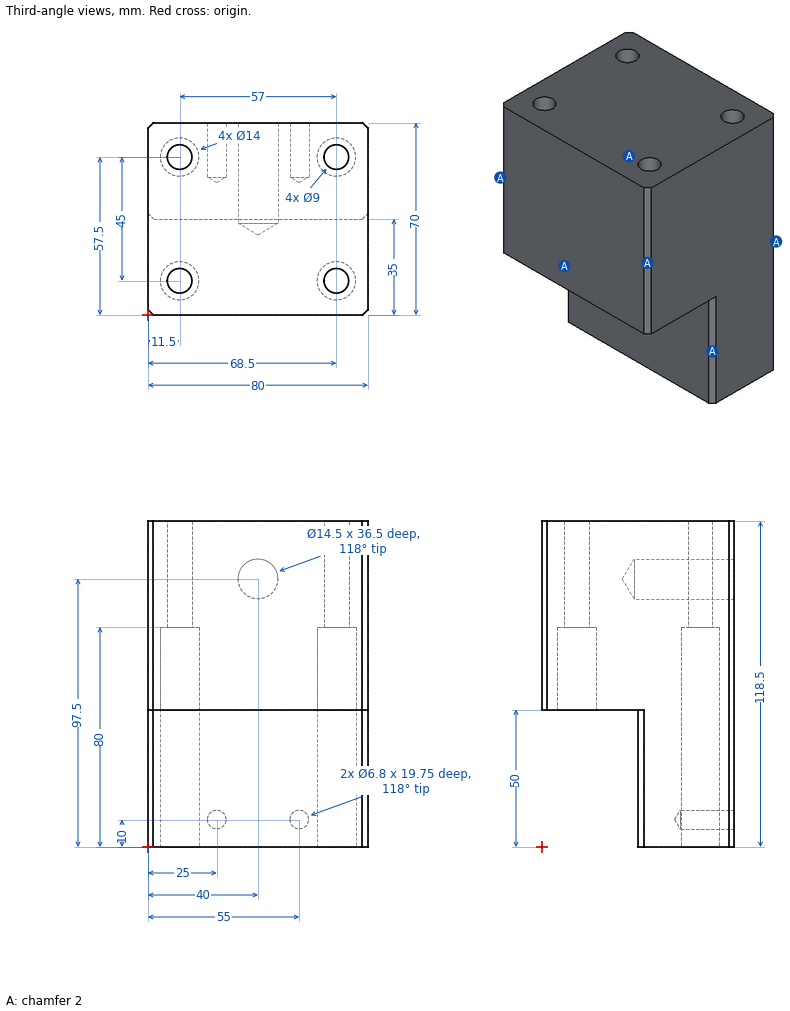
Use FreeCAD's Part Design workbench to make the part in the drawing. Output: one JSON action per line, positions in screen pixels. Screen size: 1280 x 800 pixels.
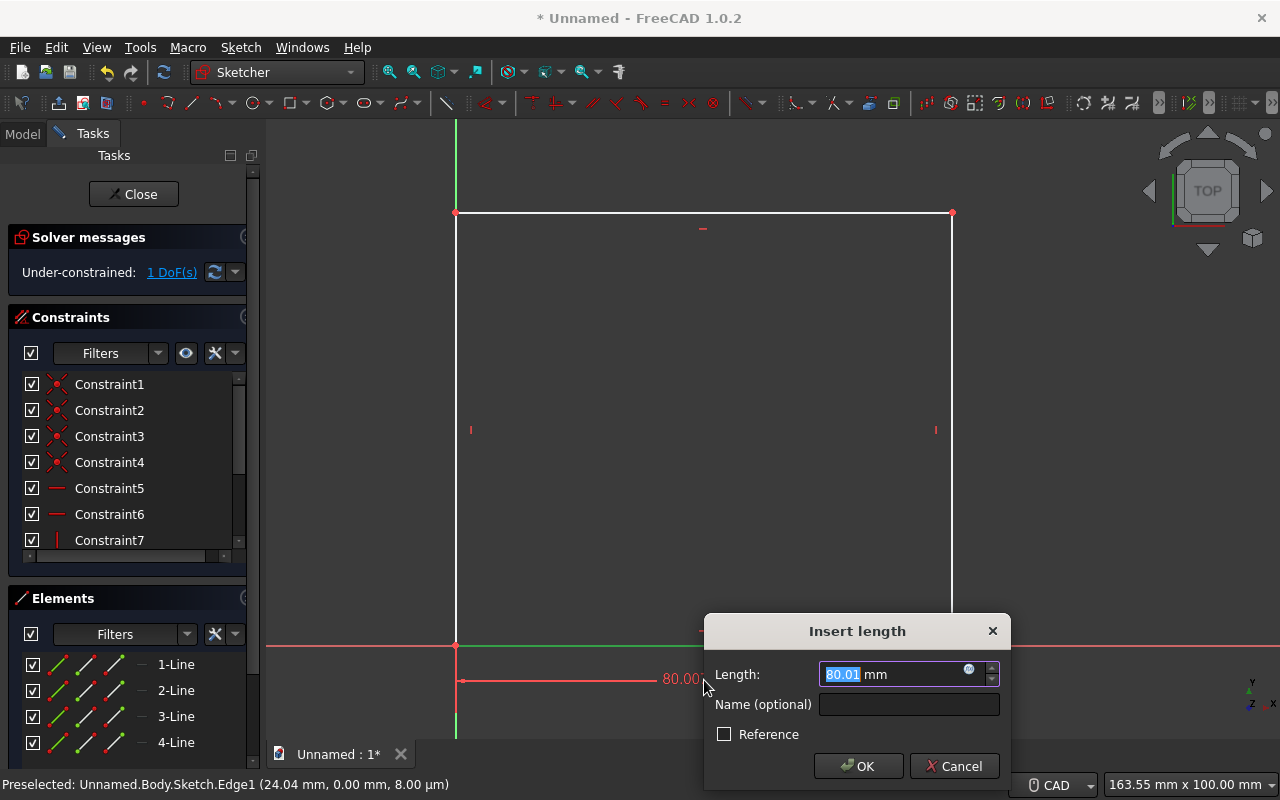
{"action": "type", "text": "80"}
{"action": "key", "text": "Return"}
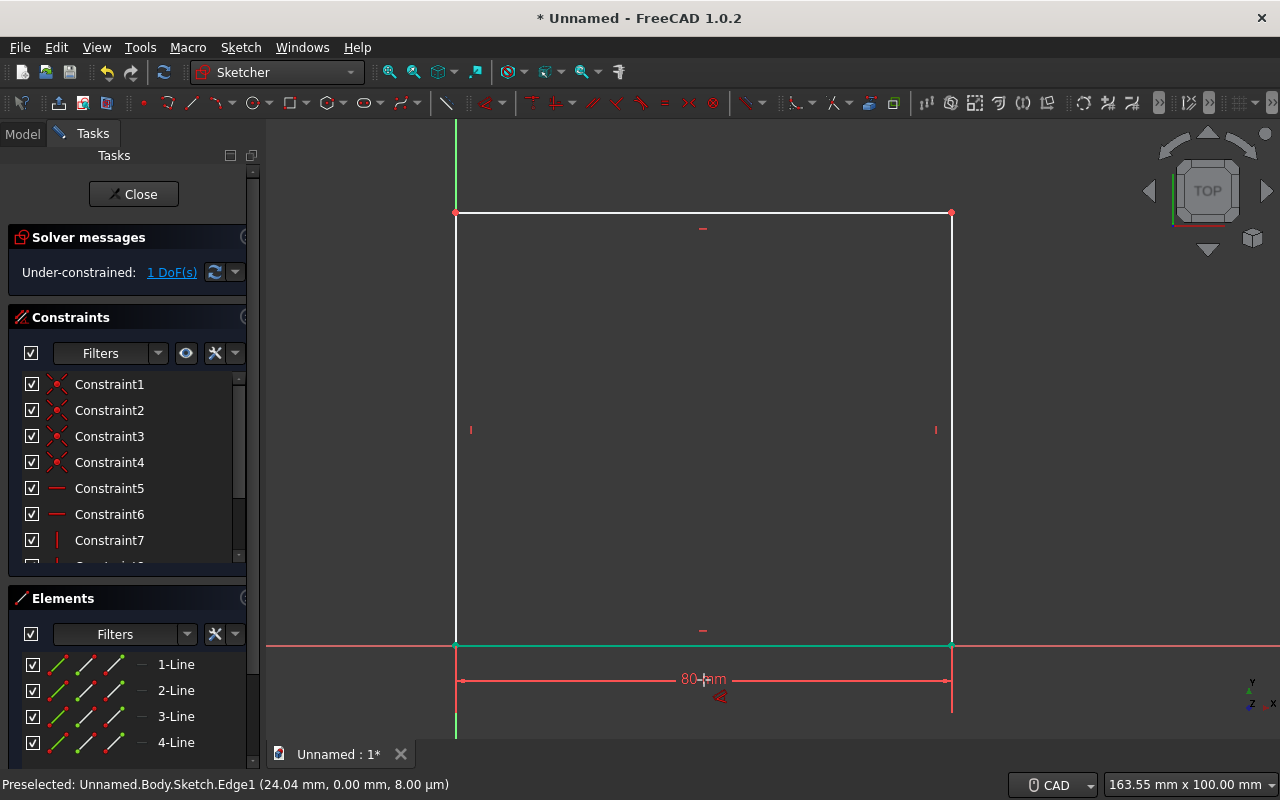
{"action": "left_click", "coordinate": [952, 516]}
{"action": "left_click", "coordinate": [986, 429]}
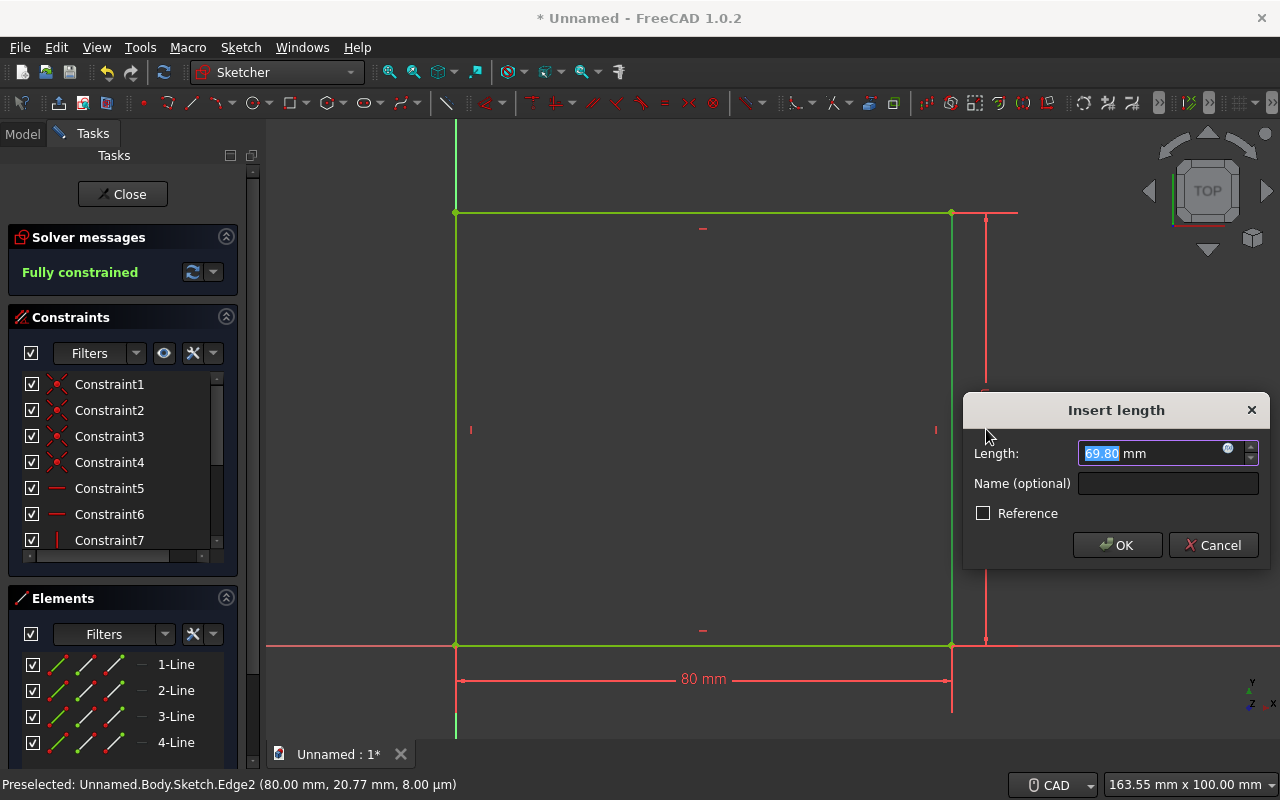
{"action": "type", "text": "70"}
{"action": "key", "text": "Return"}
{"action": "key", "text": "Escape"}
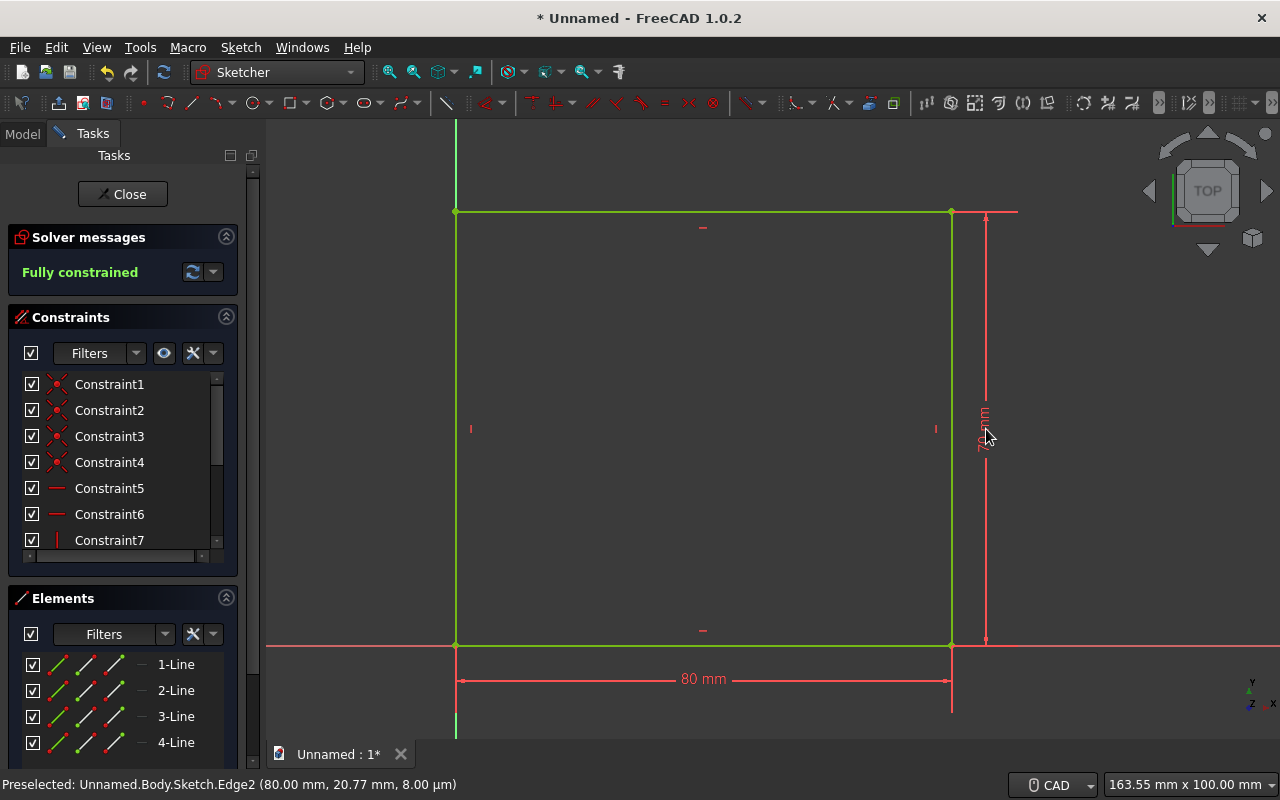
{"action": "left_click", "coordinate": [123, 194]}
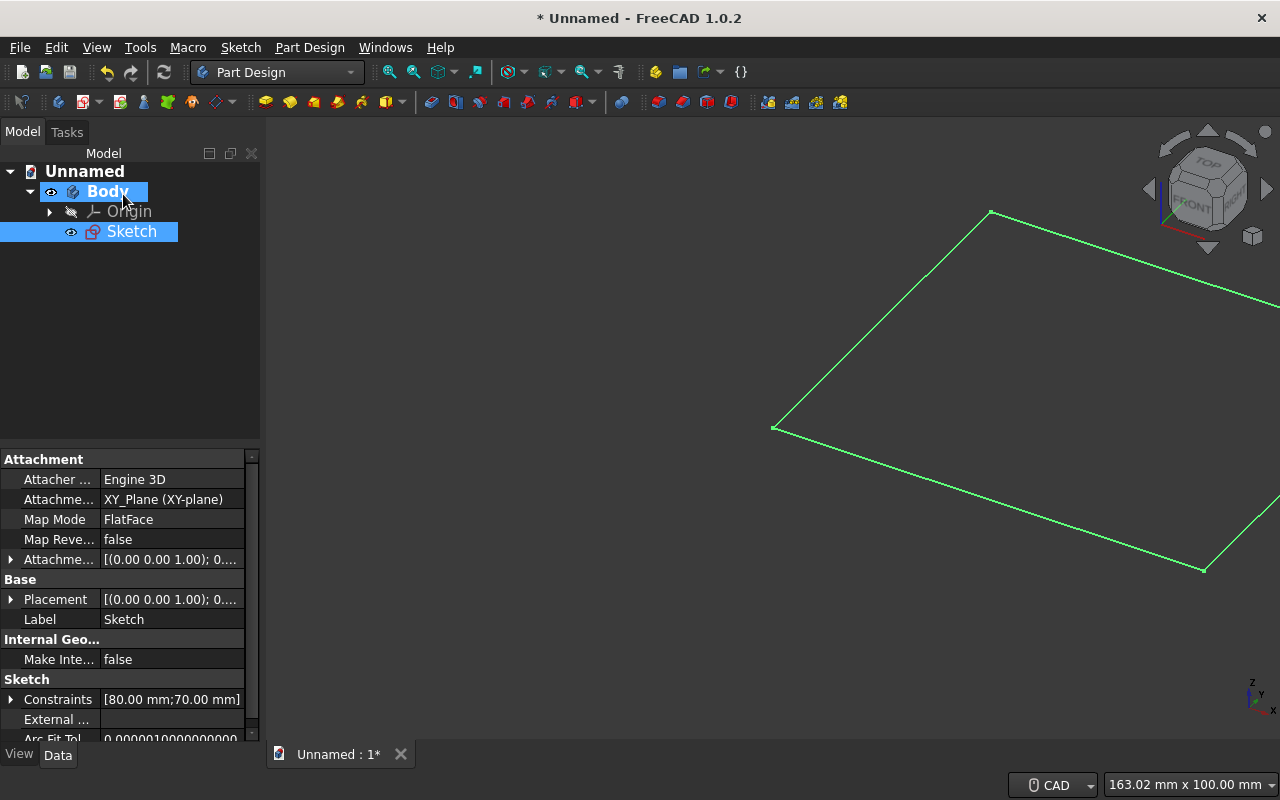
{"action": "left_click", "coordinate": [266, 102]}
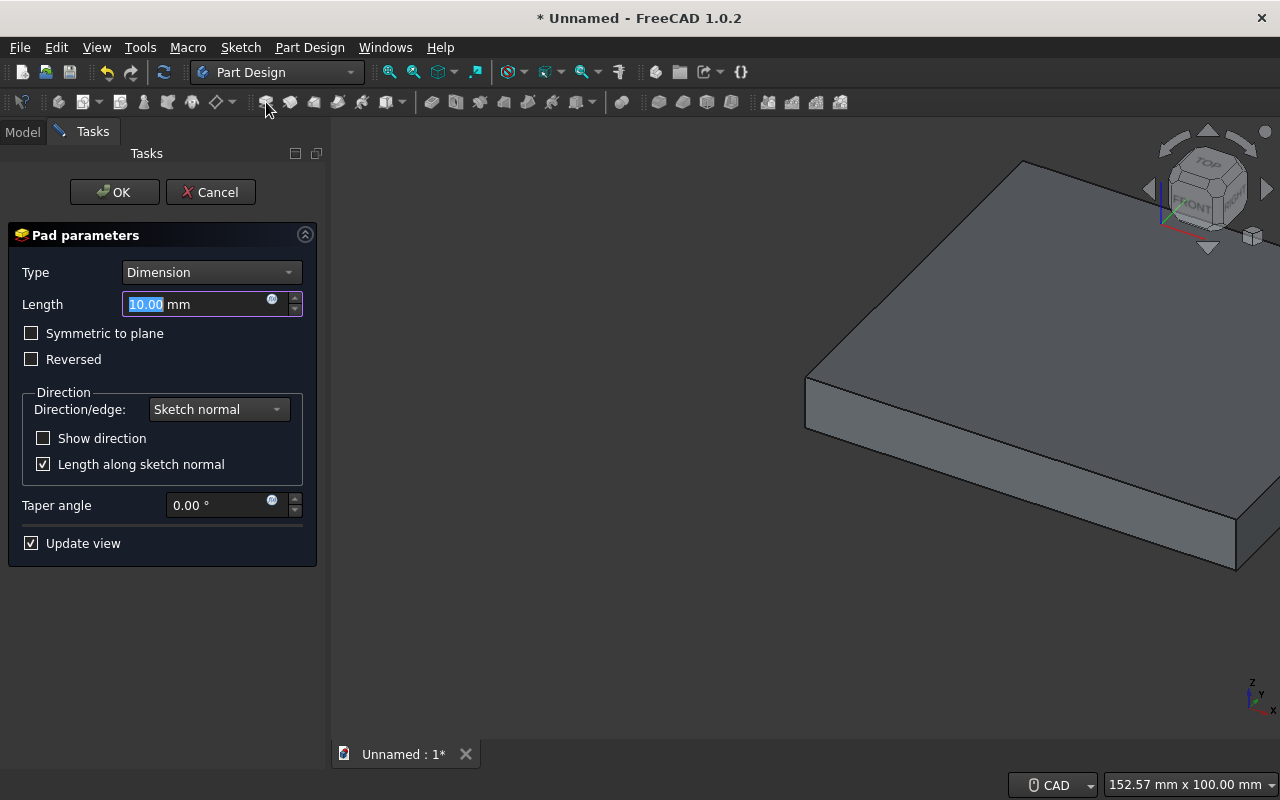
{"action": "type", "text": "118.5"}
{"action": "key", "text": "Tab"}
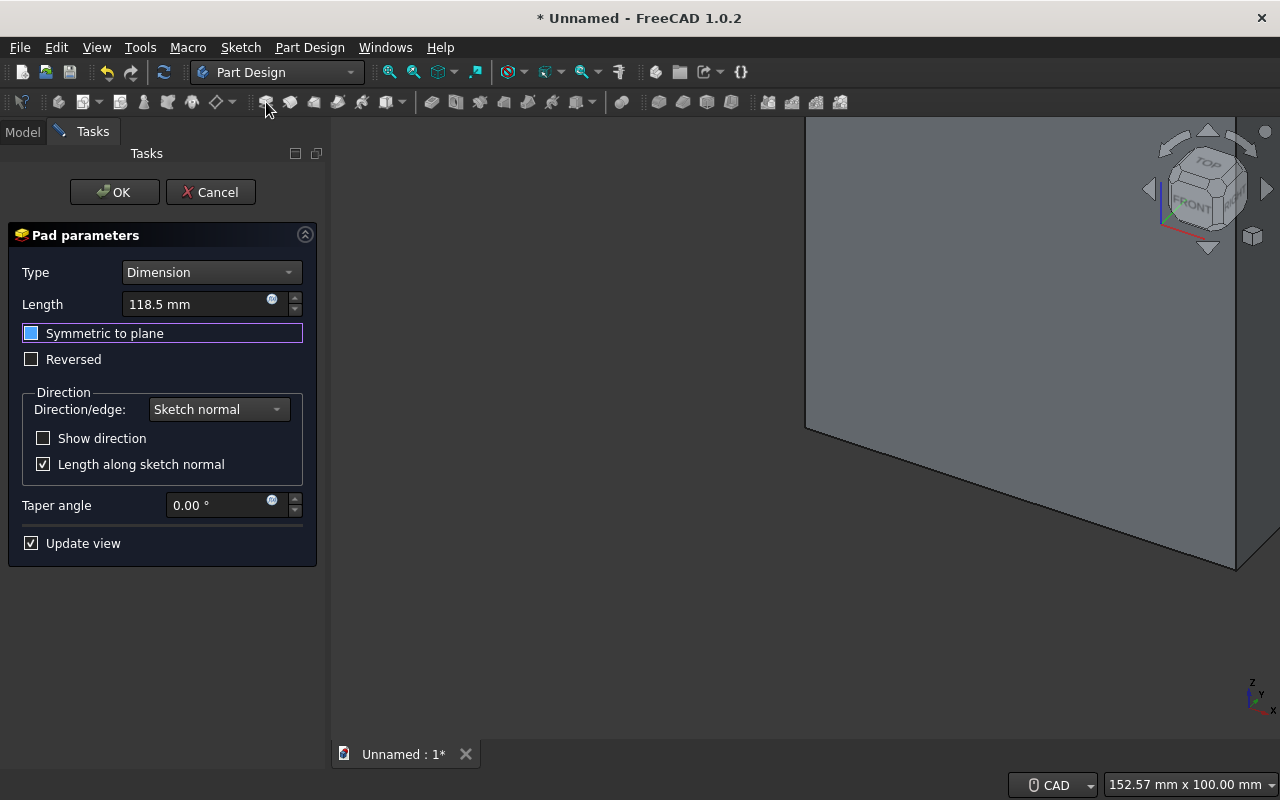
{"action": "left_click", "coordinate": [115, 192]}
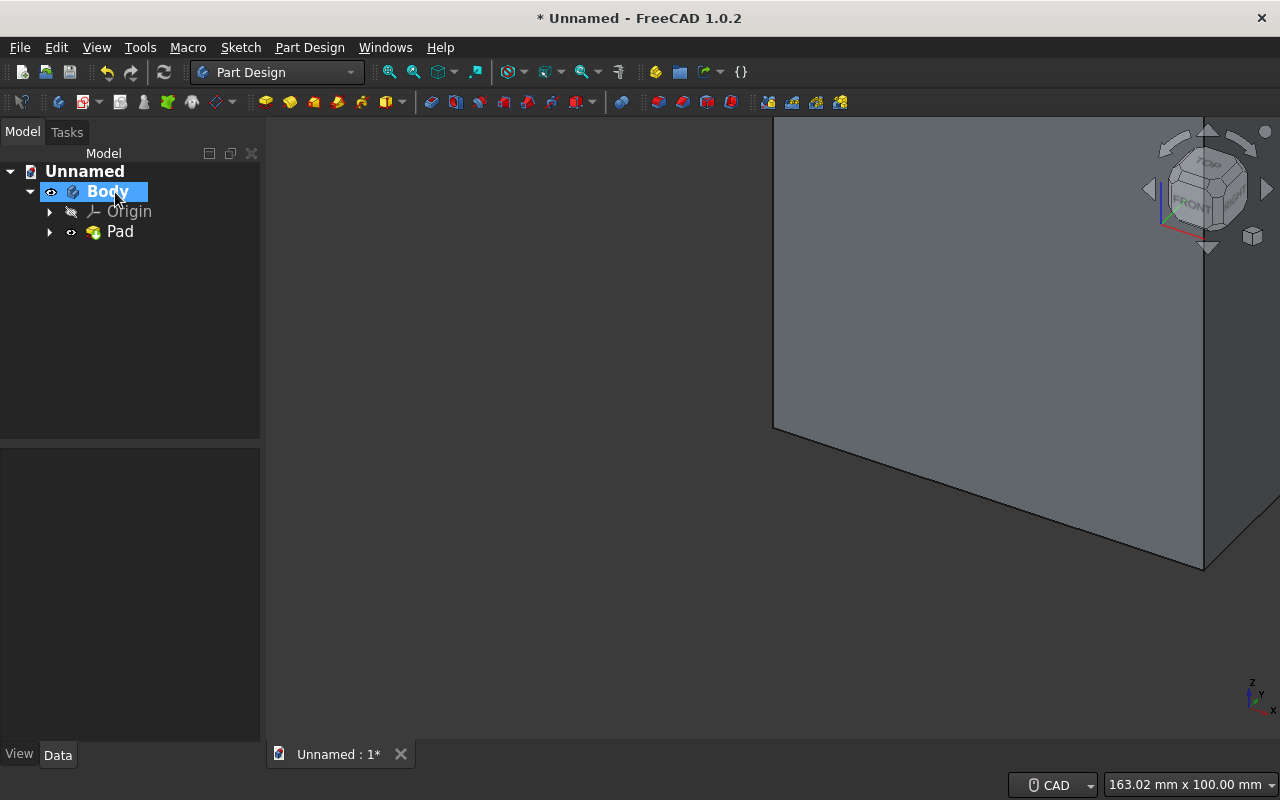
{"action": "key", "text": "v f"}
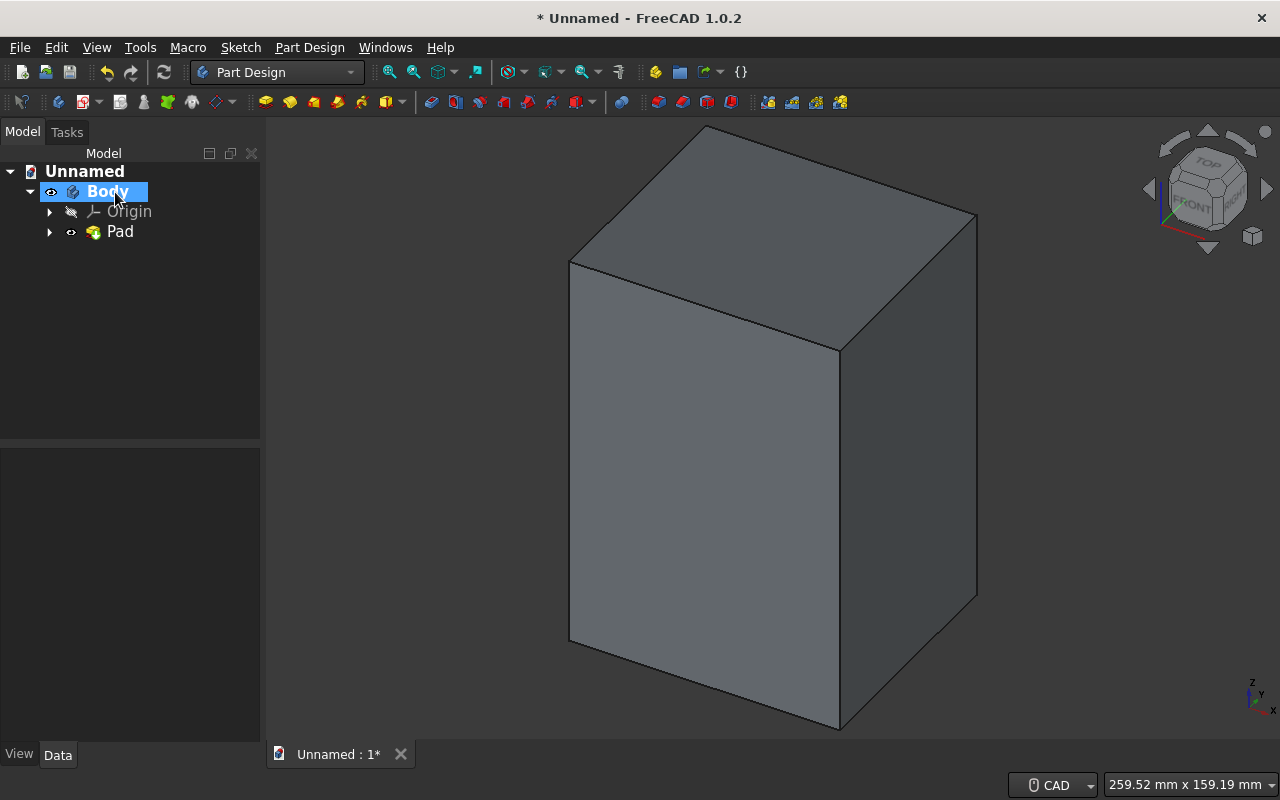
{"action": "left_click", "coordinate": [84, 102]}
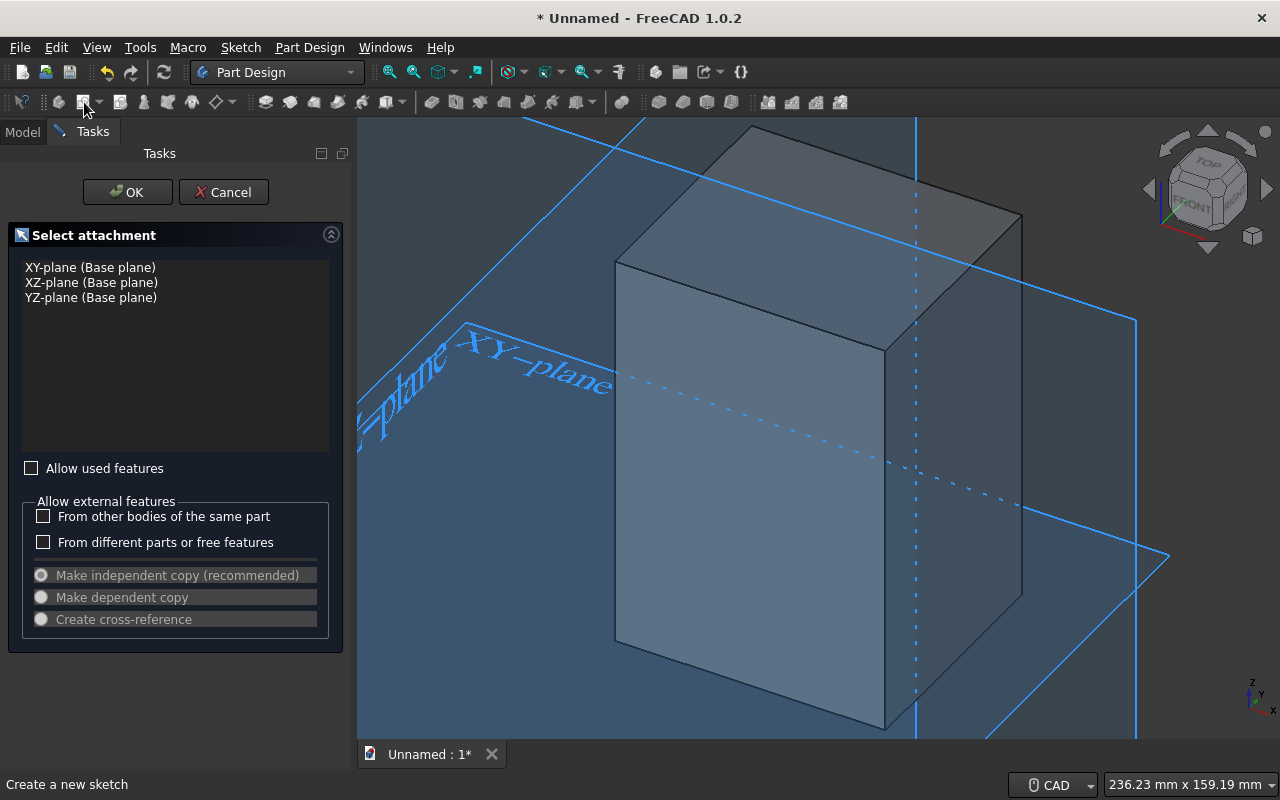
{"action": "left_click", "coordinate": [82, 268]}